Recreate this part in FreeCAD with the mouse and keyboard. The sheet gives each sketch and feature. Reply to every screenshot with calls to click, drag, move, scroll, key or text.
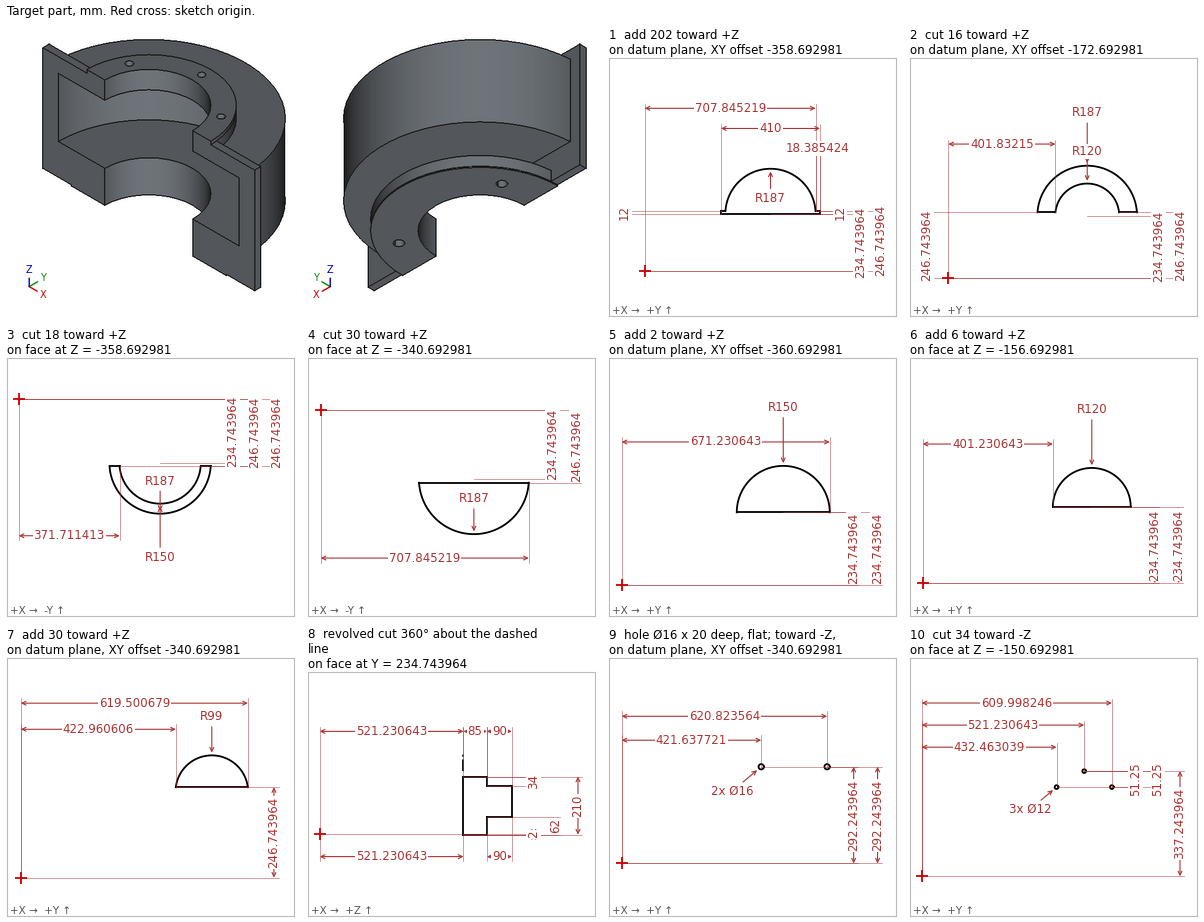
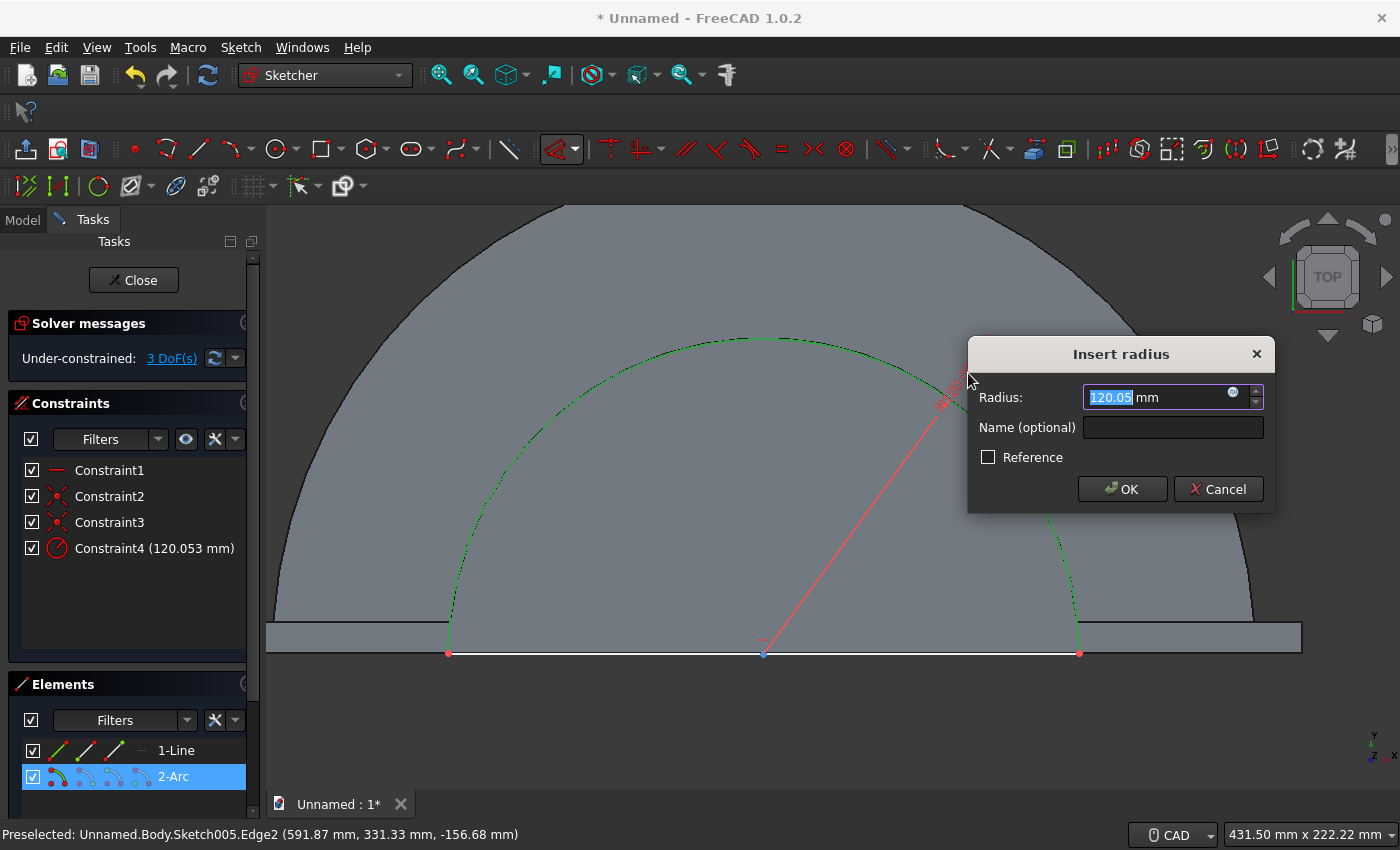
text(120)
key(Return)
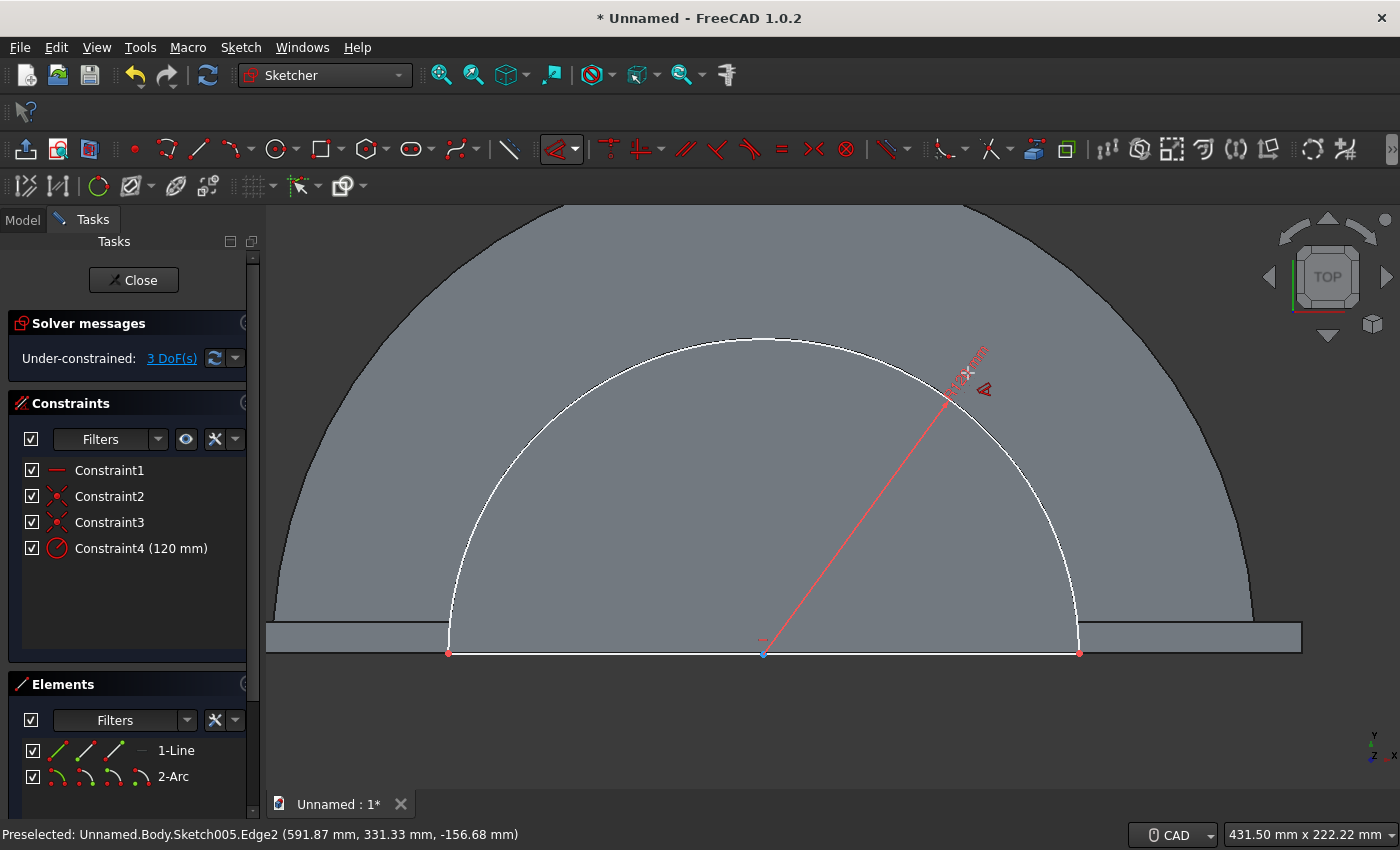
click(448, 654)
click(371, 620)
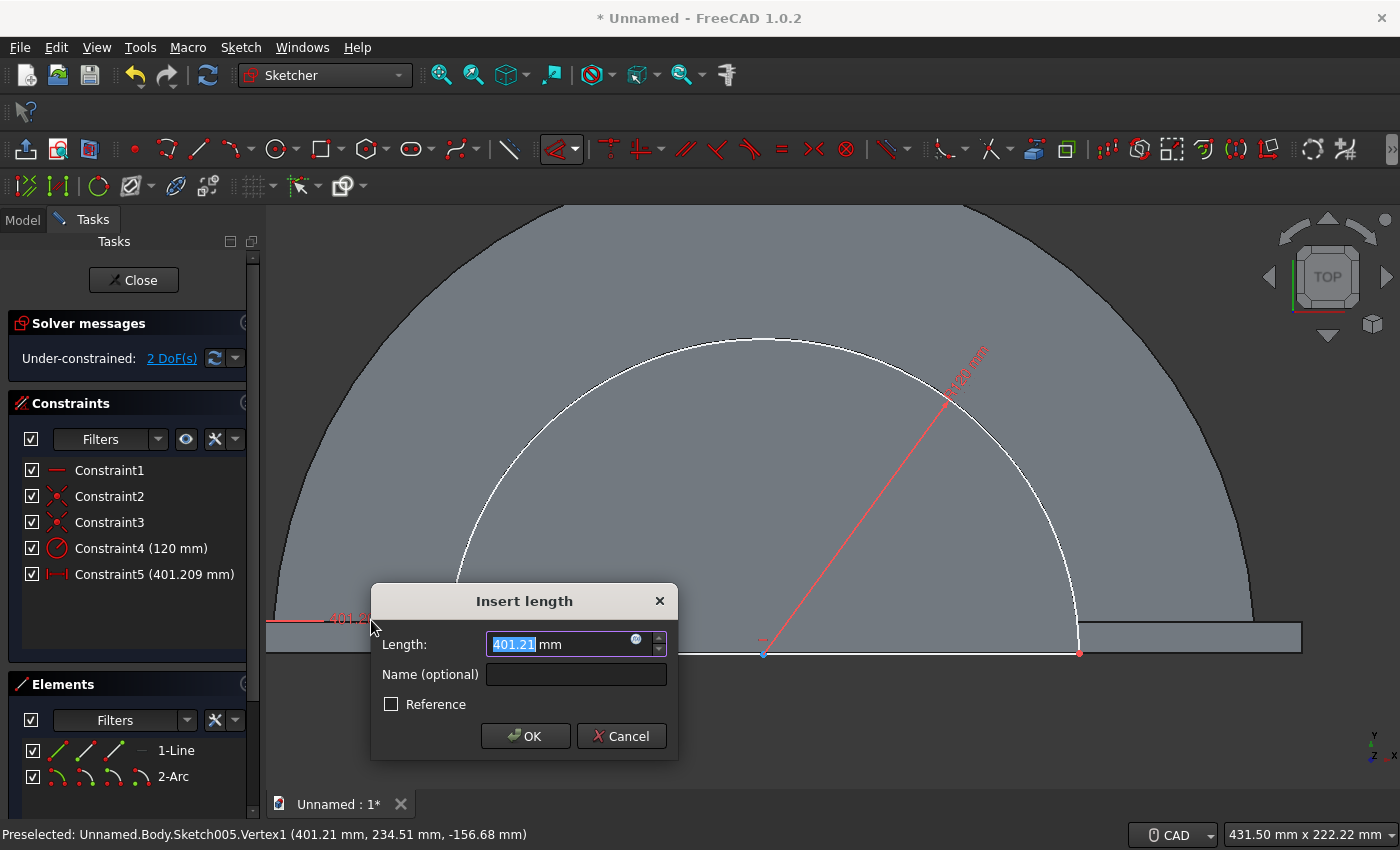
text(401.230643)
key(Return)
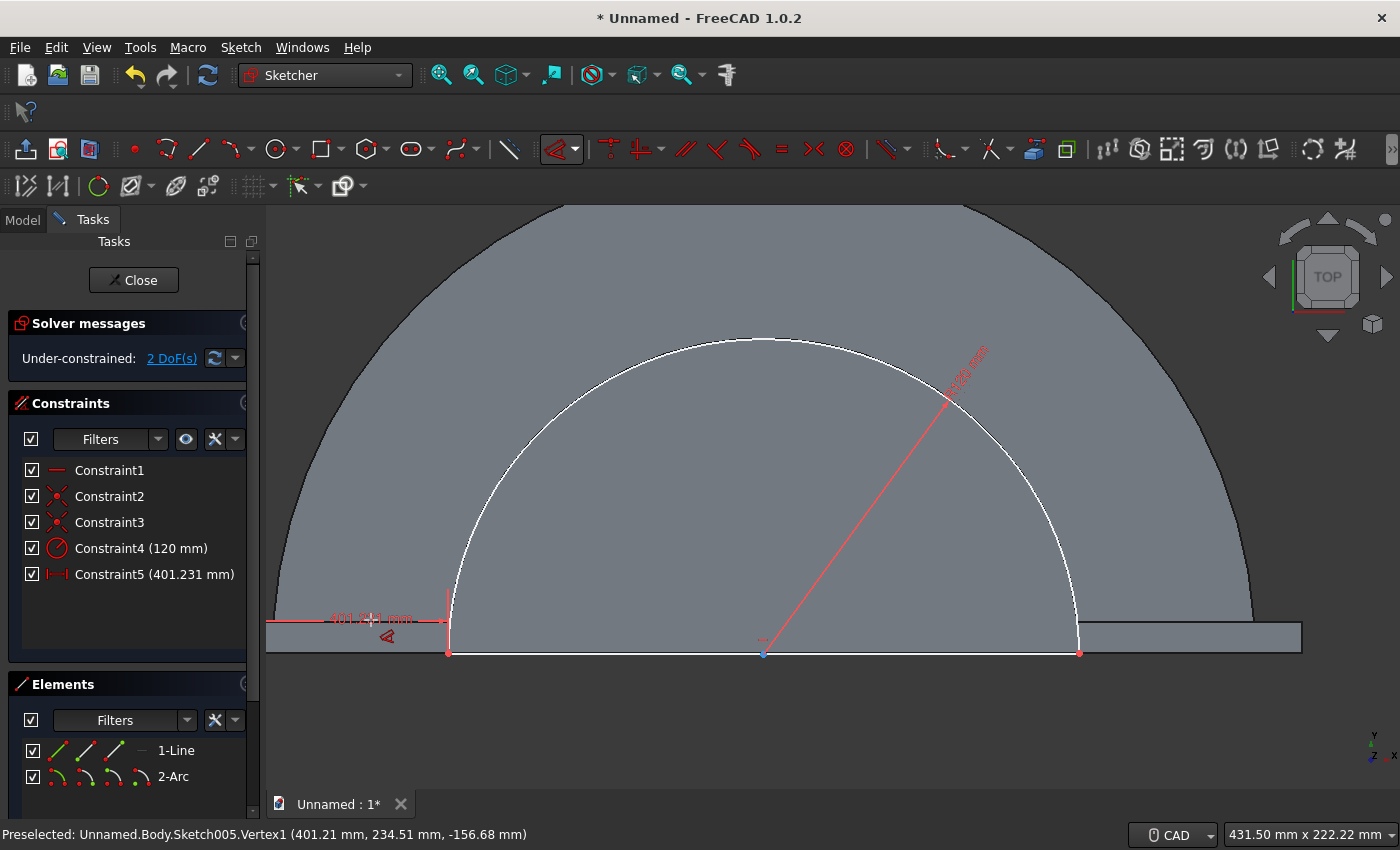
click(448, 654)
click(482, 708)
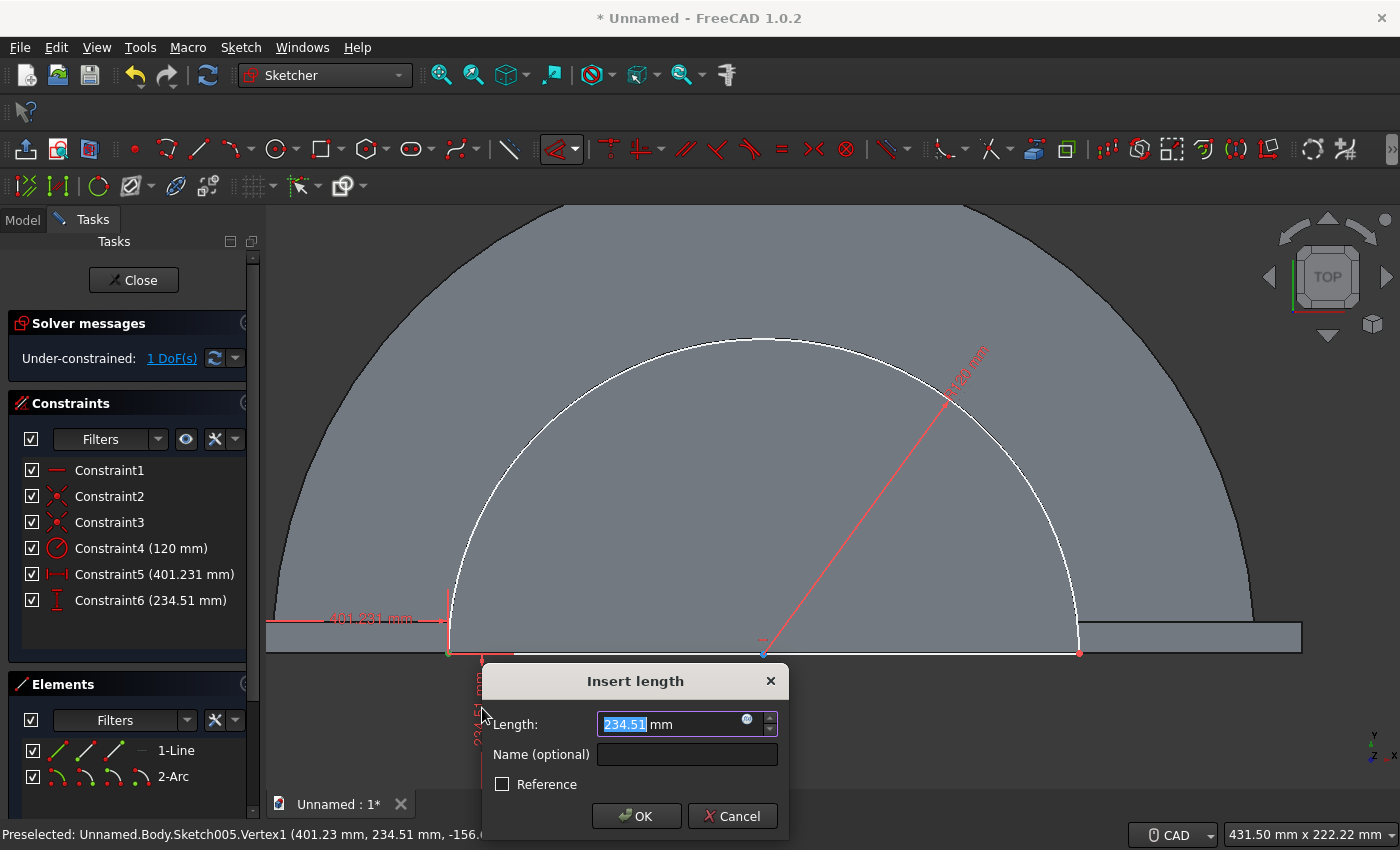
text(234.743964)
key(Return)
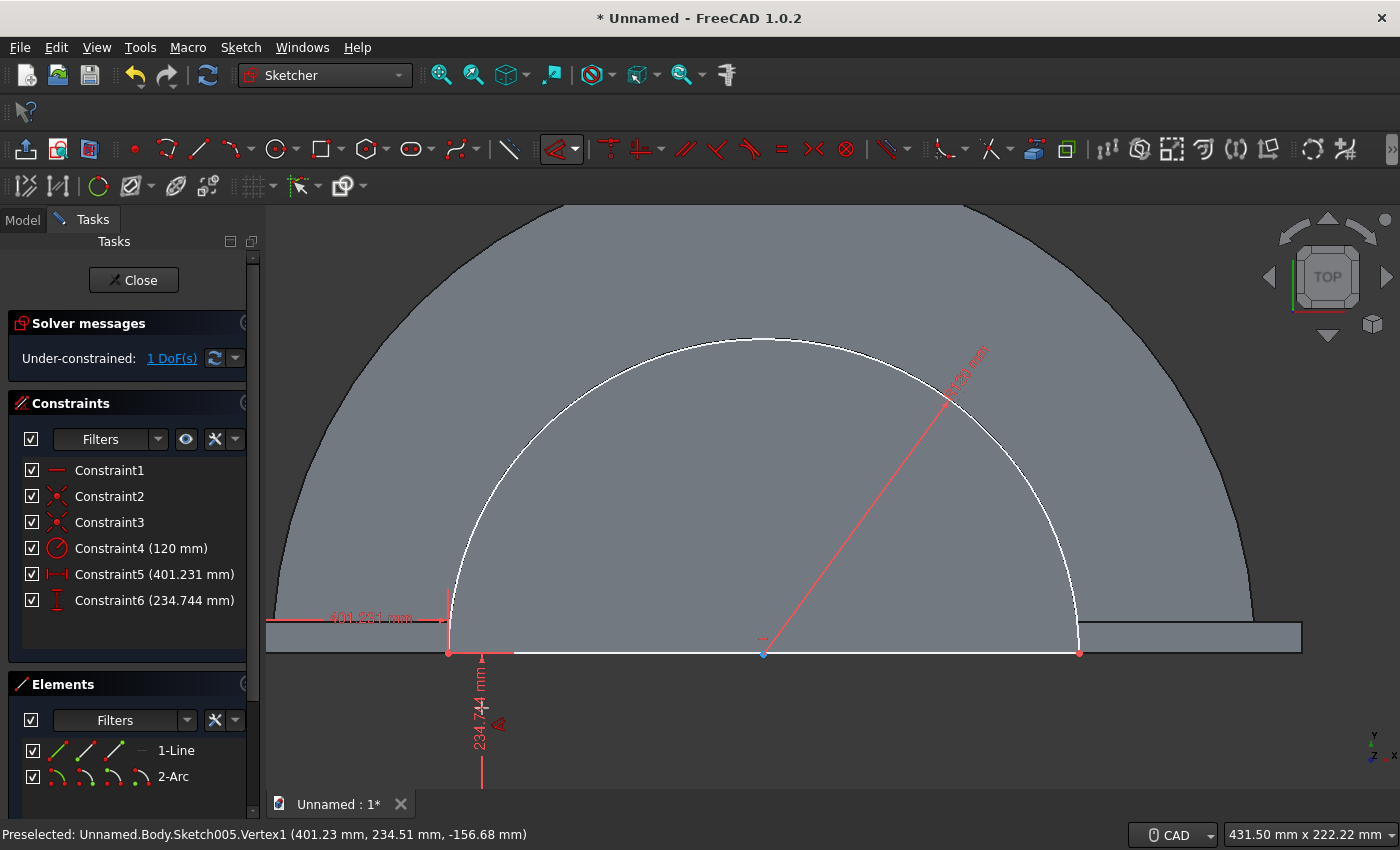
click(764, 655)
click(798, 708)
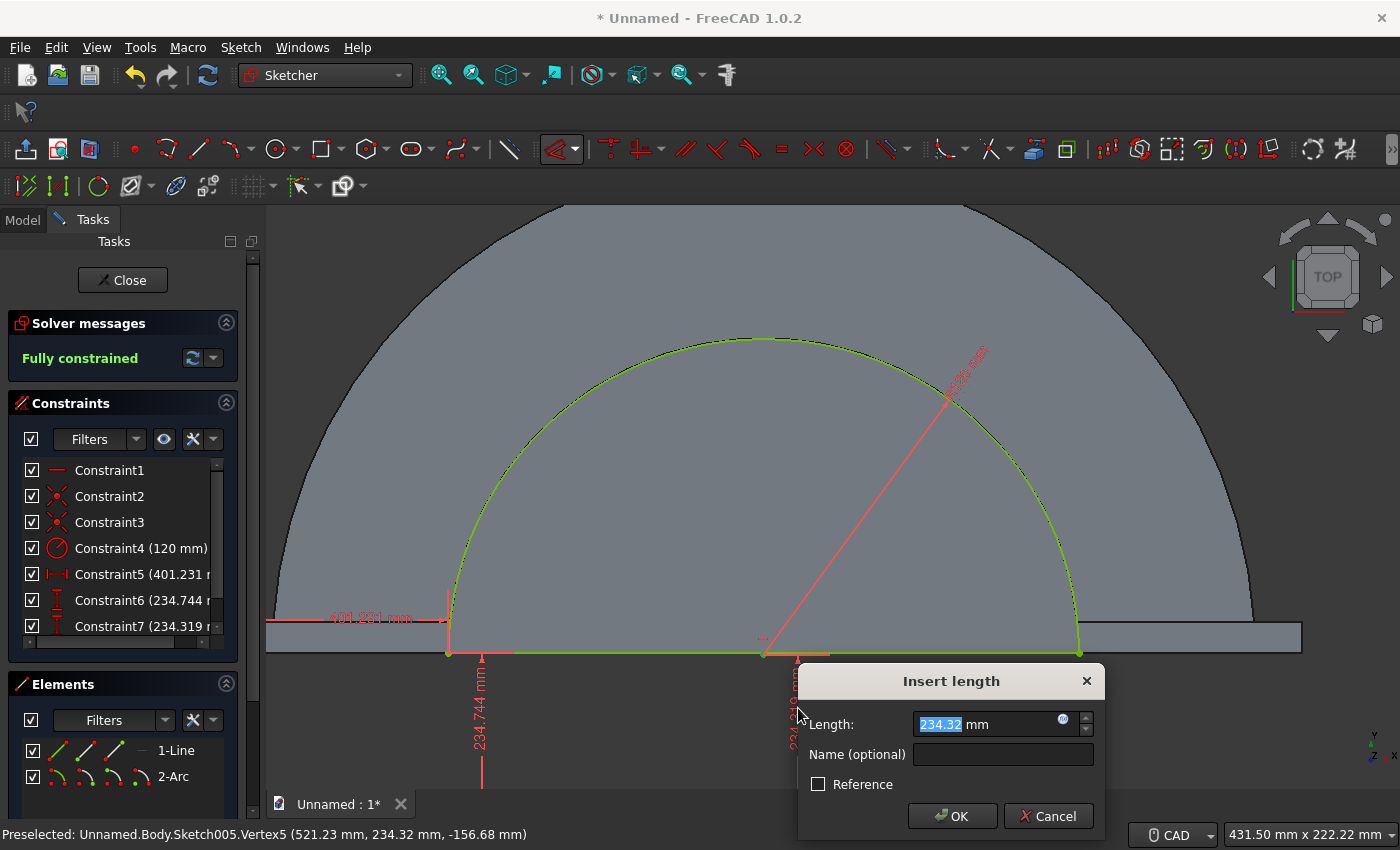
text(234.743964)
key(Return)
key(Escape)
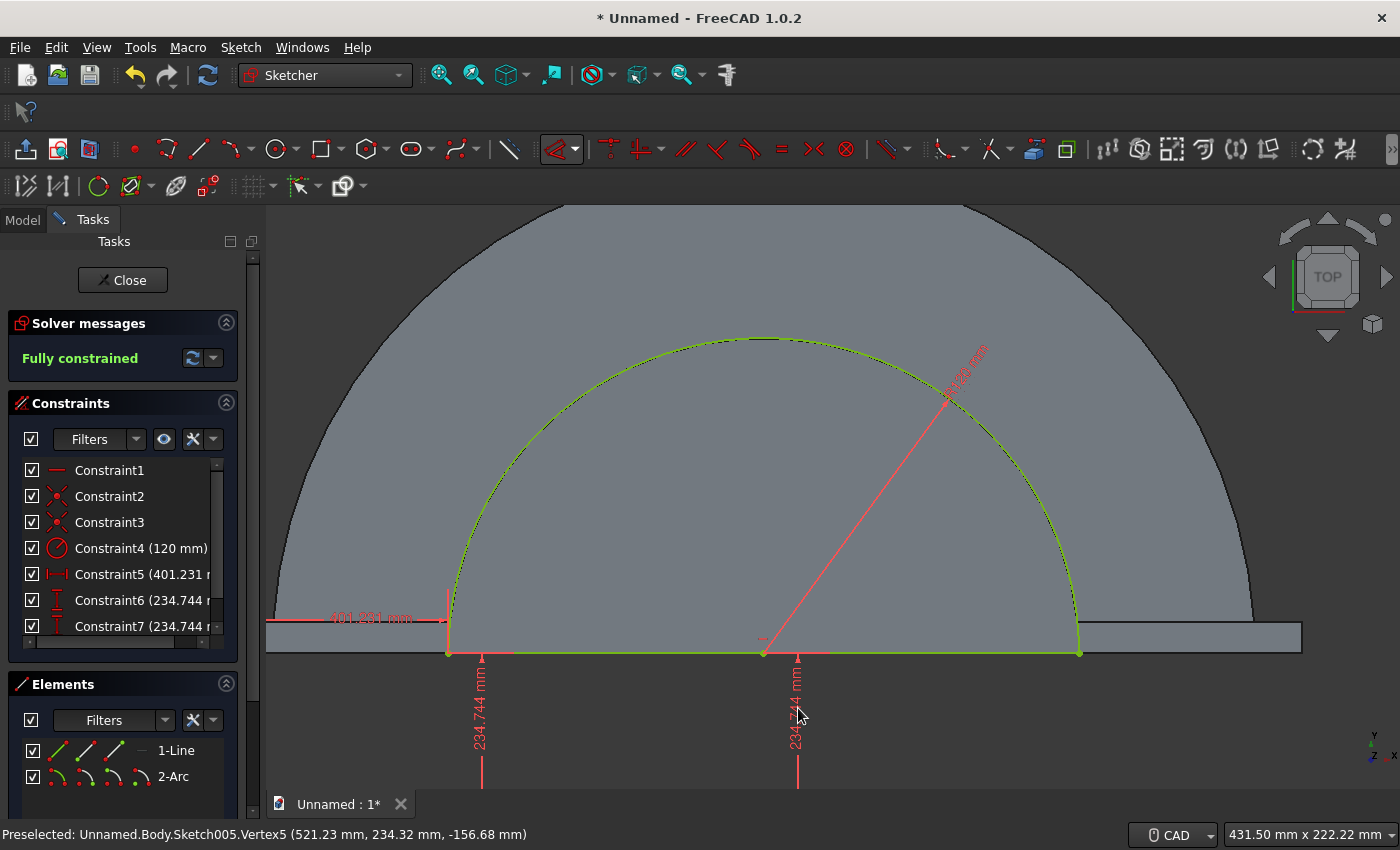
click(123, 280)